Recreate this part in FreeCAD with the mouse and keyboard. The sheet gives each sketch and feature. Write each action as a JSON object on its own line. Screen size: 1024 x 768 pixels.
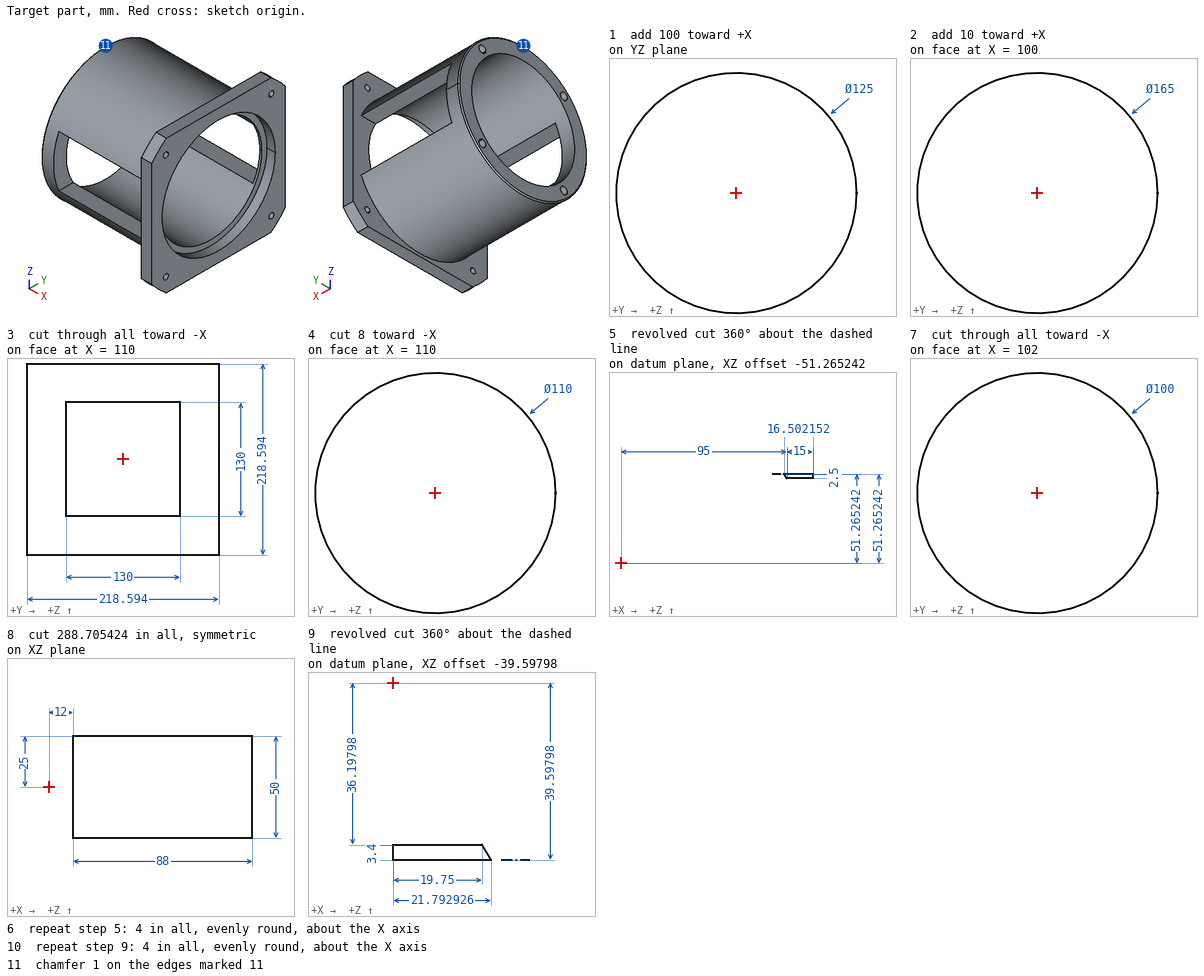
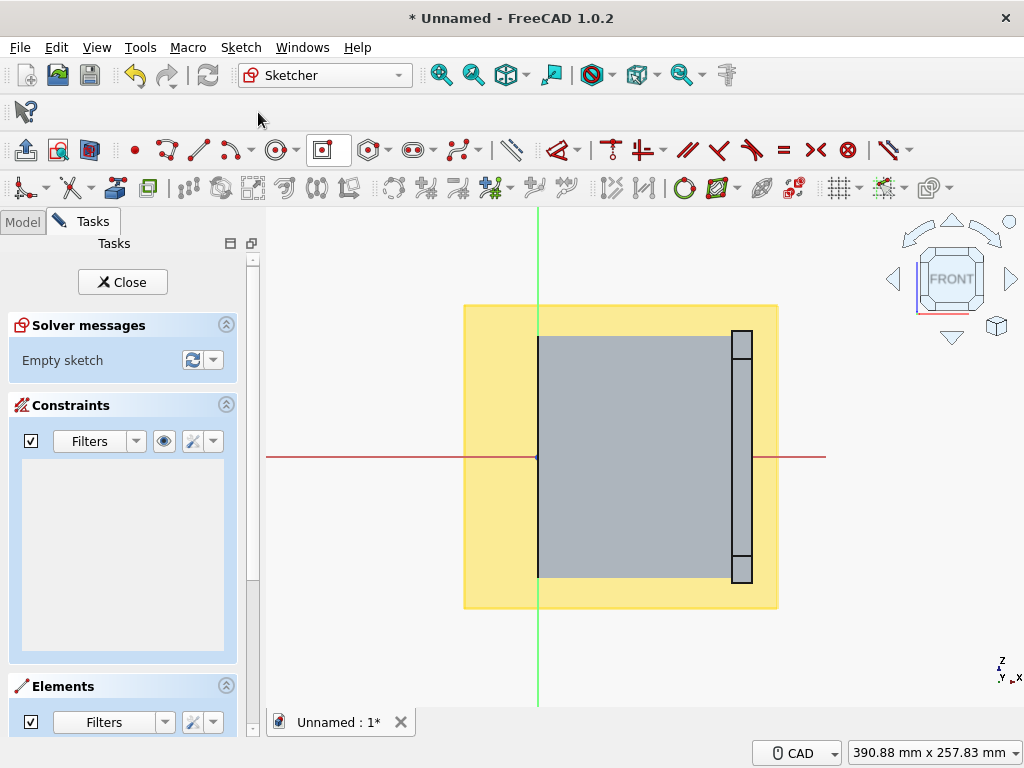
{"action": "left_click", "coordinate": [90, 150]}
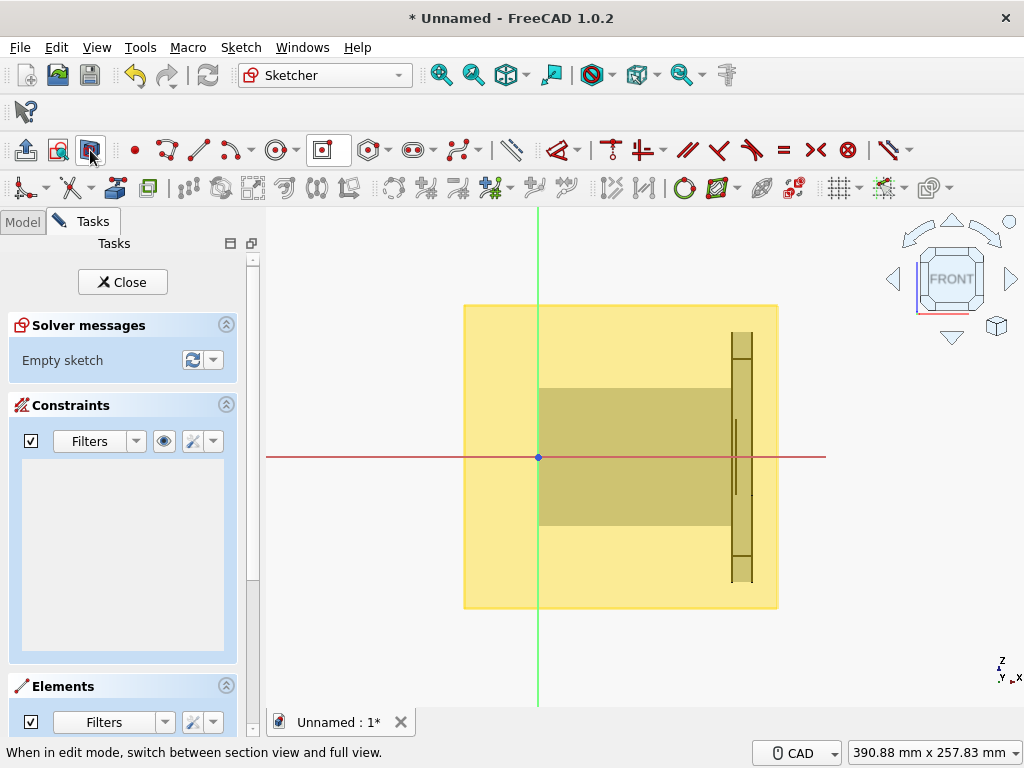
{"action": "scroll", "coordinate": [748, 348], "scroll_direction": "up", "scroll_amount": 11}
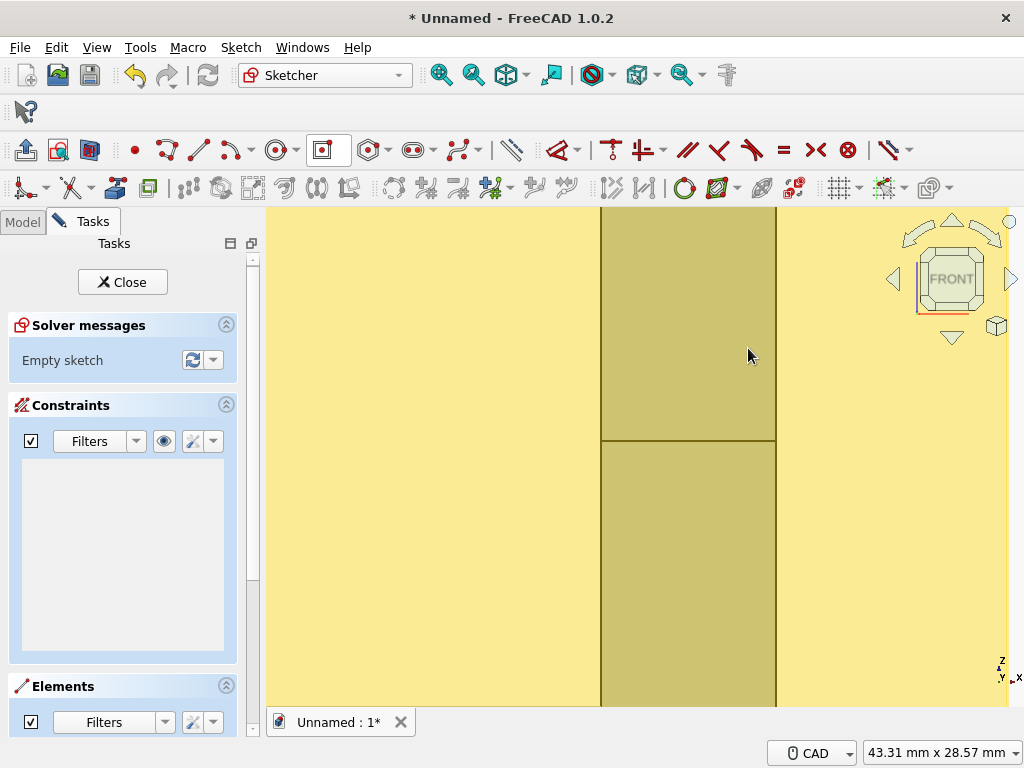
{"action": "left_click", "coordinate": [168, 150]}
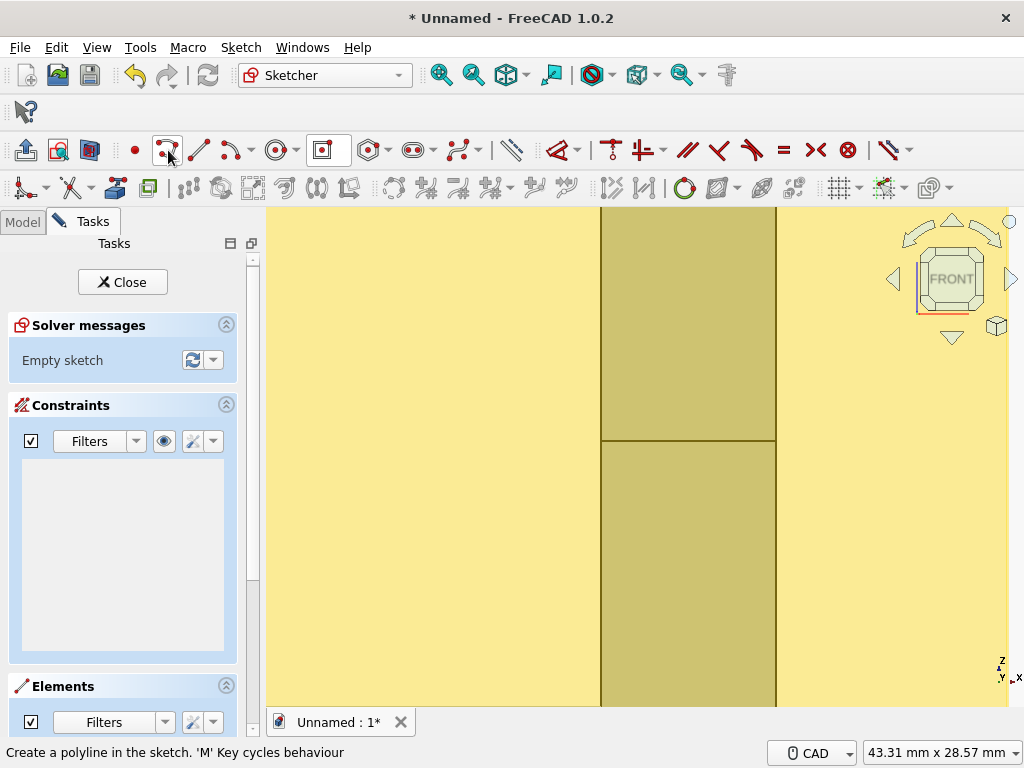
{"action": "left_click", "coordinate": [487, 433]}
{"action": "left_click", "coordinate": [776, 433]}
{"action": "left_click", "coordinate": [776, 477]}
{"action": "left_click", "coordinate": [513, 477]}
{"action": "left_click", "coordinate": [487, 434]}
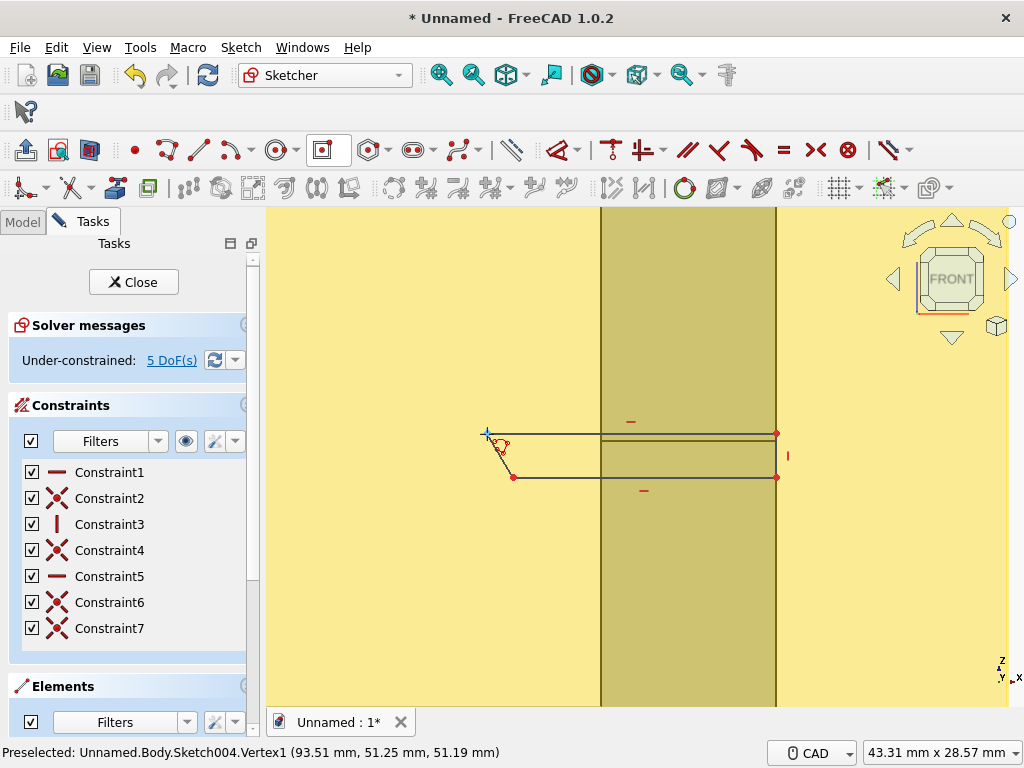
{"action": "left_click", "coordinate": [200, 150]}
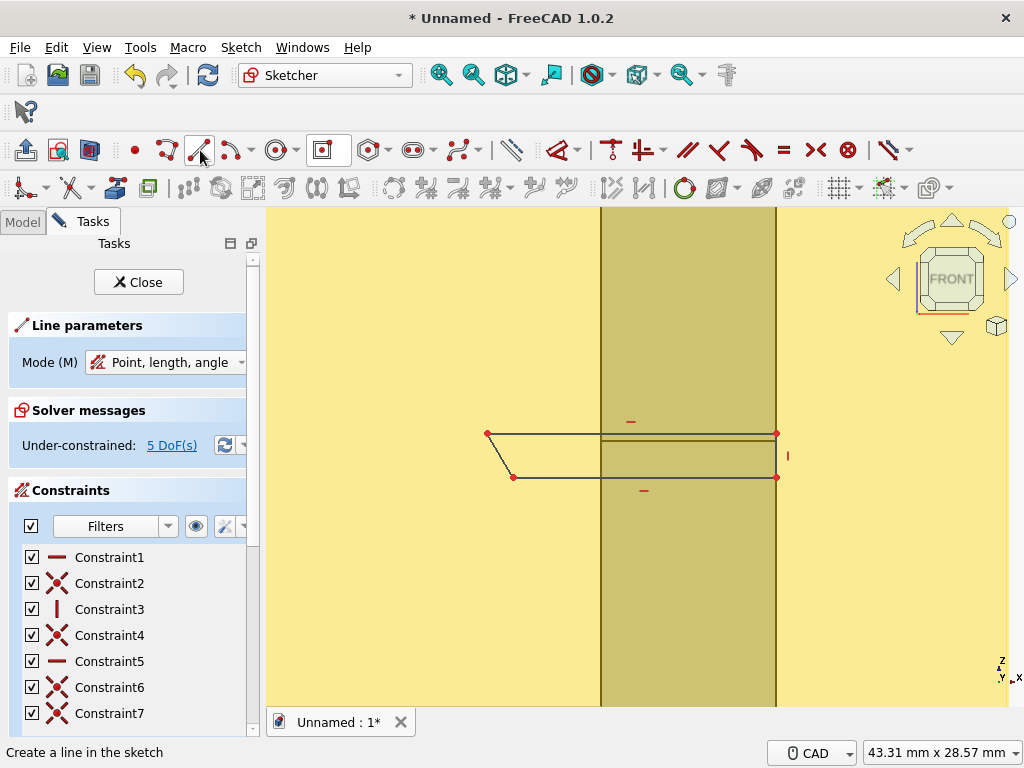
{"action": "left_click", "coordinate": [458, 433]}
{"action": "left_click", "coordinate": [371, 433]}
{"action": "key", "text": "Escape"}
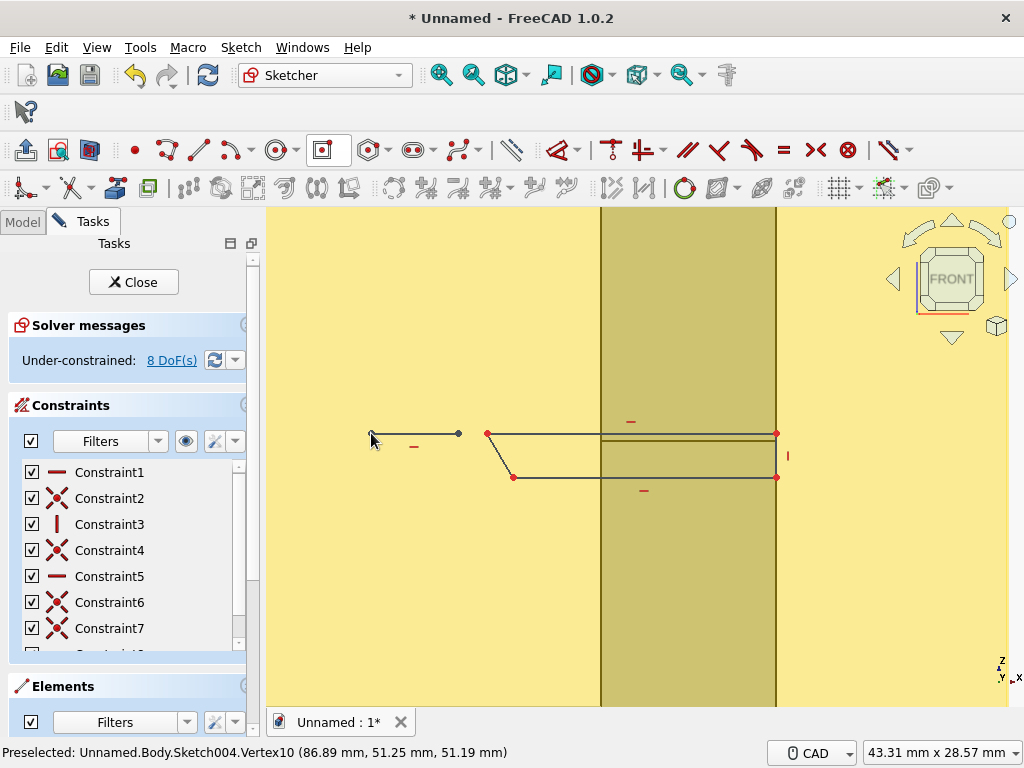
{"action": "left_click", "coordinate": [432, 434]}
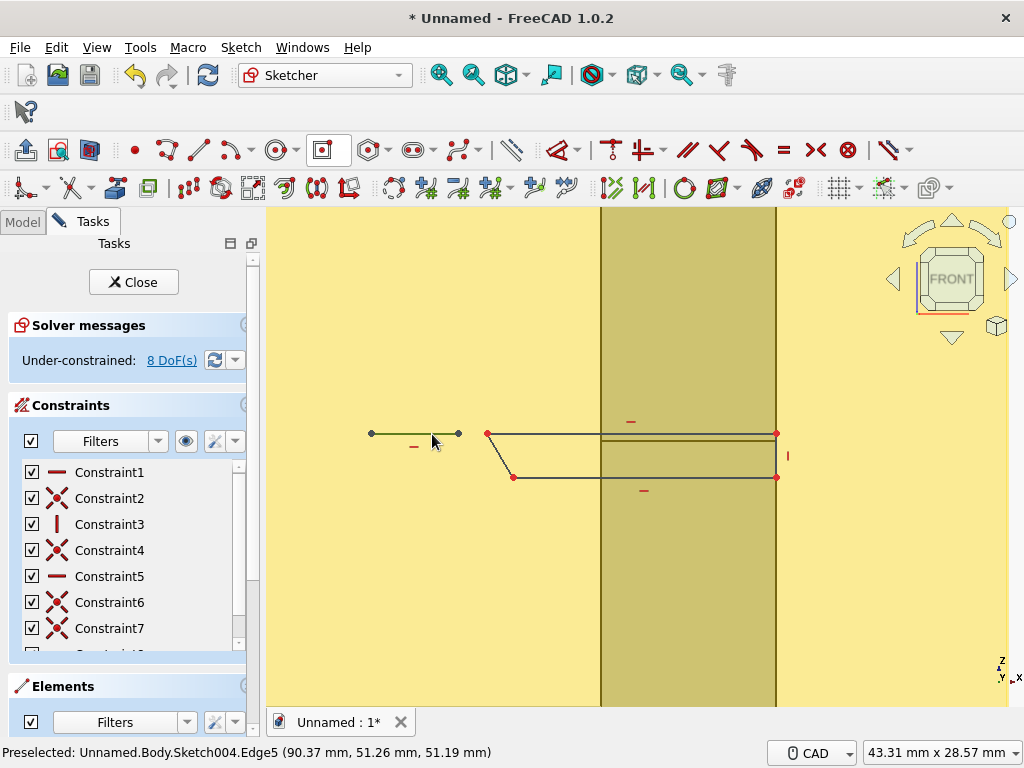
{"action": "left_click", "coordinate": [512, 150]}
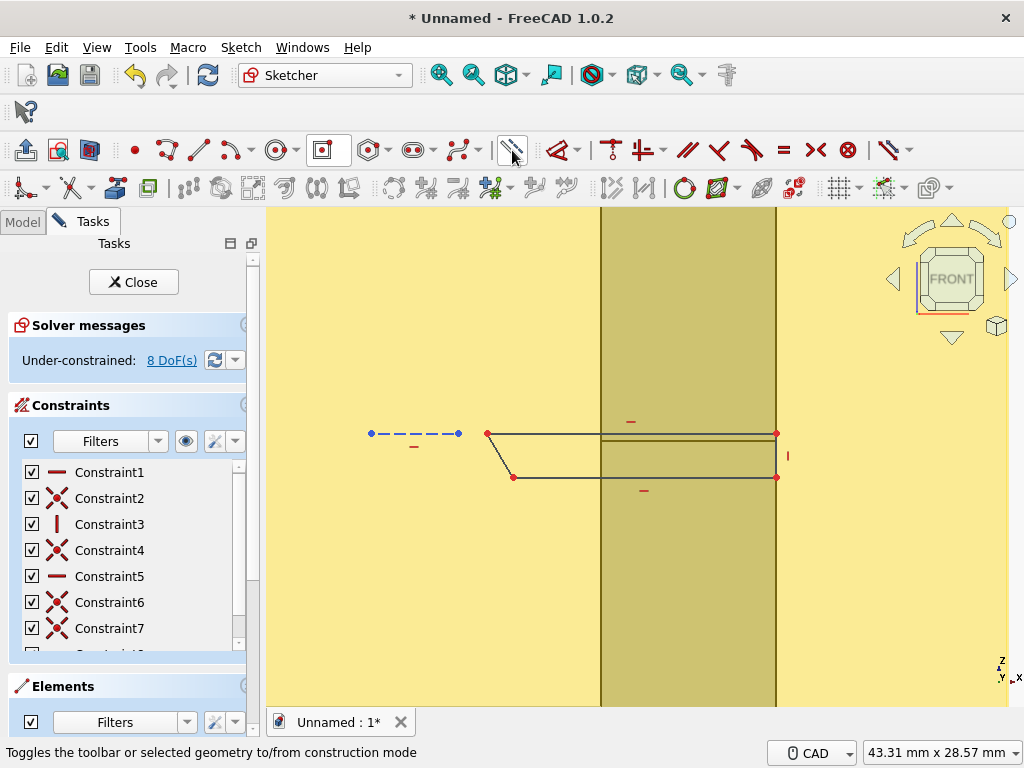
{"action": "left_click", "coordinate": [558, 150]}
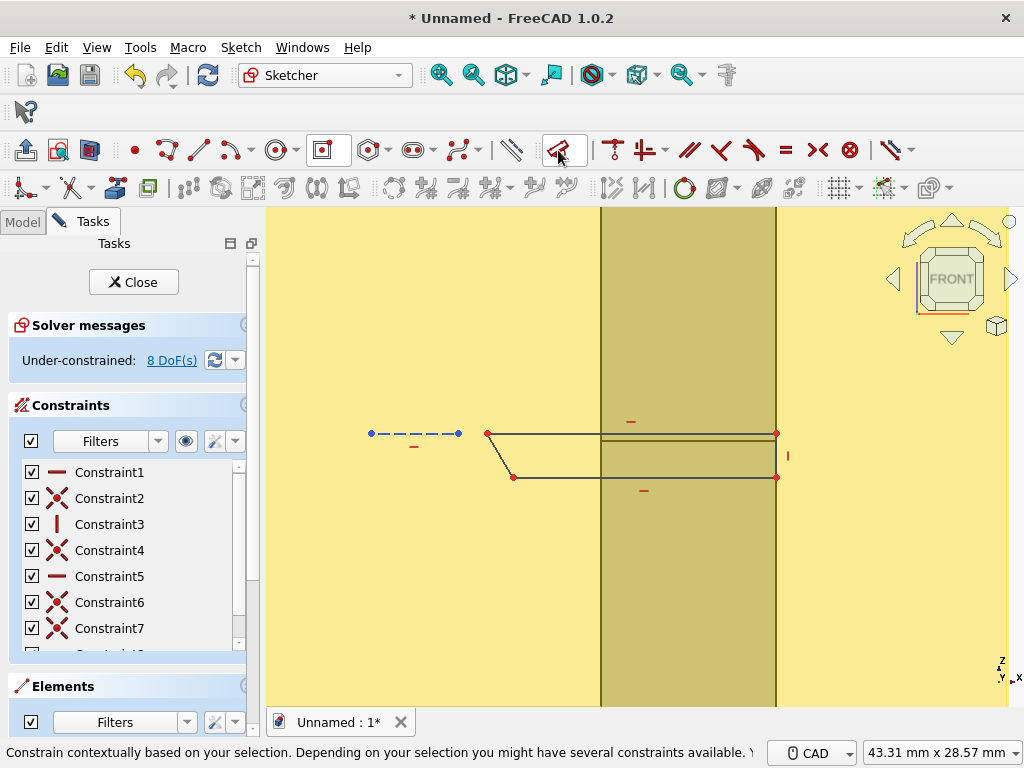
{"action": "left_click", "coordinate": [697, 478]}
{"action": "left_click", "coordinate": [645, 512]}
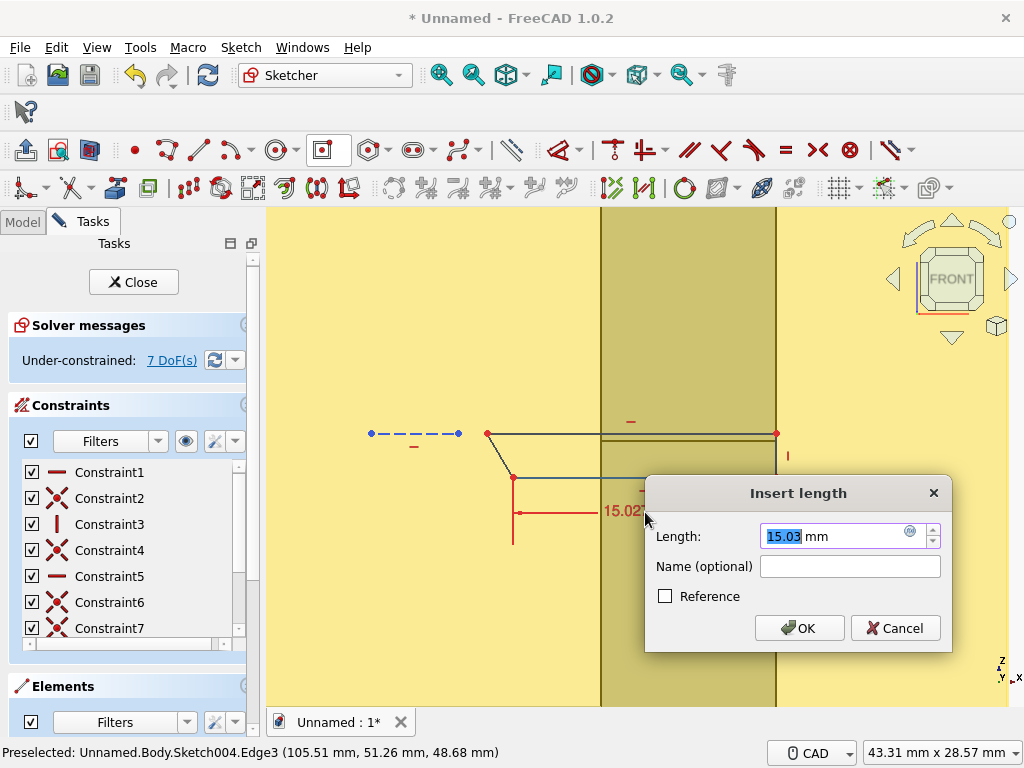
{"action": "type", "text": "15"}
{"action": "key", "text": "Return"}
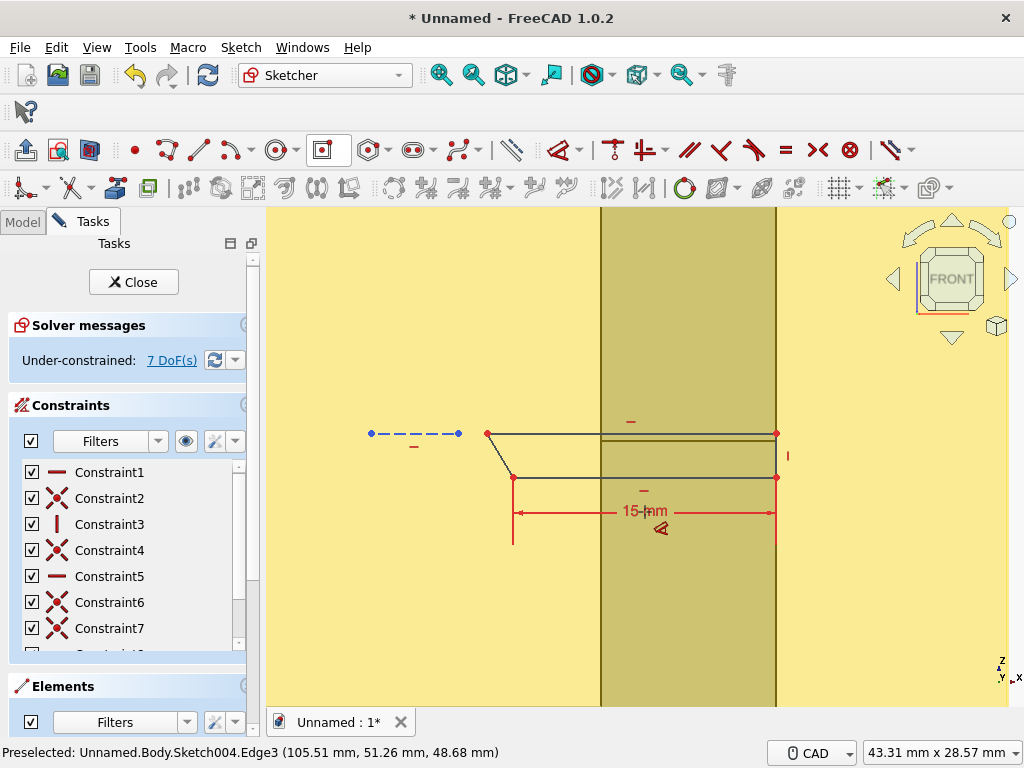
{"action": "left_click", "coordinate": [776, 447]}
{"action": "left_click", "coordinate": [810, 456]}